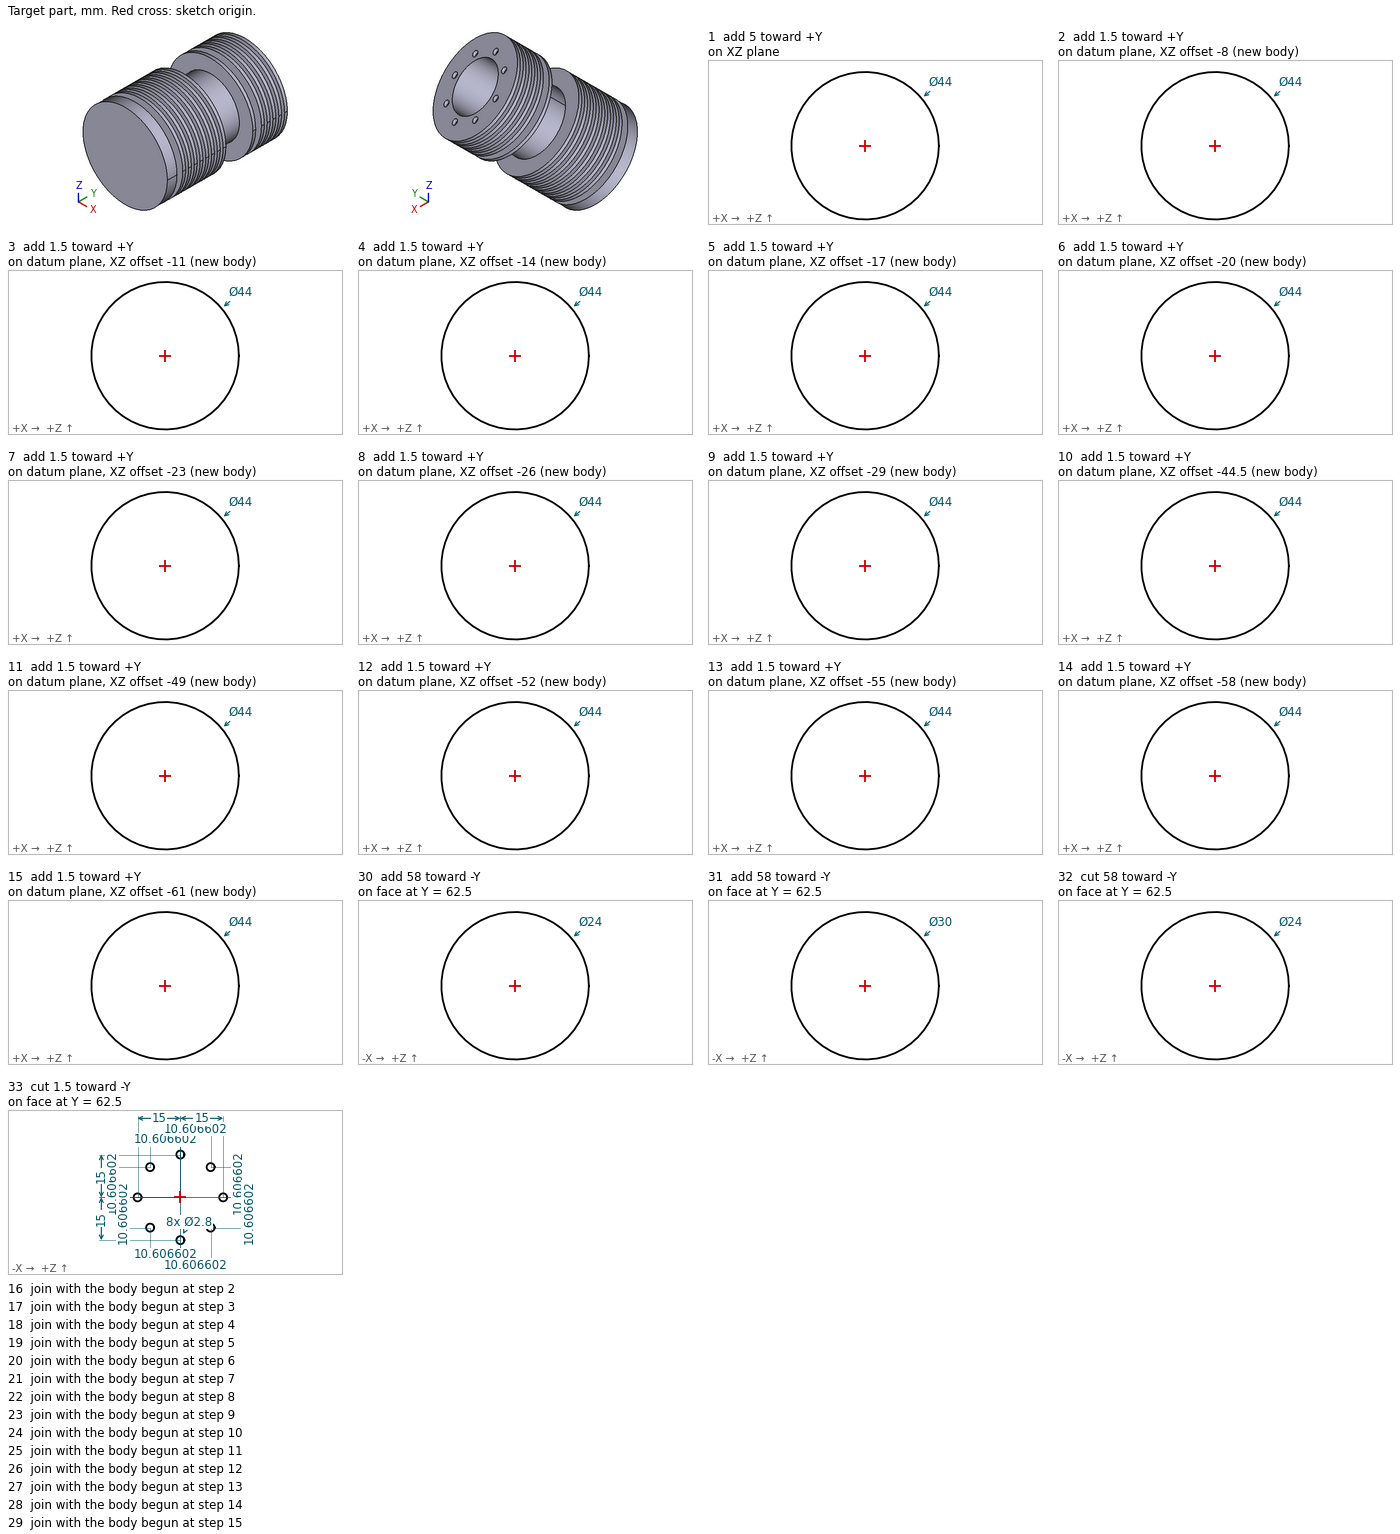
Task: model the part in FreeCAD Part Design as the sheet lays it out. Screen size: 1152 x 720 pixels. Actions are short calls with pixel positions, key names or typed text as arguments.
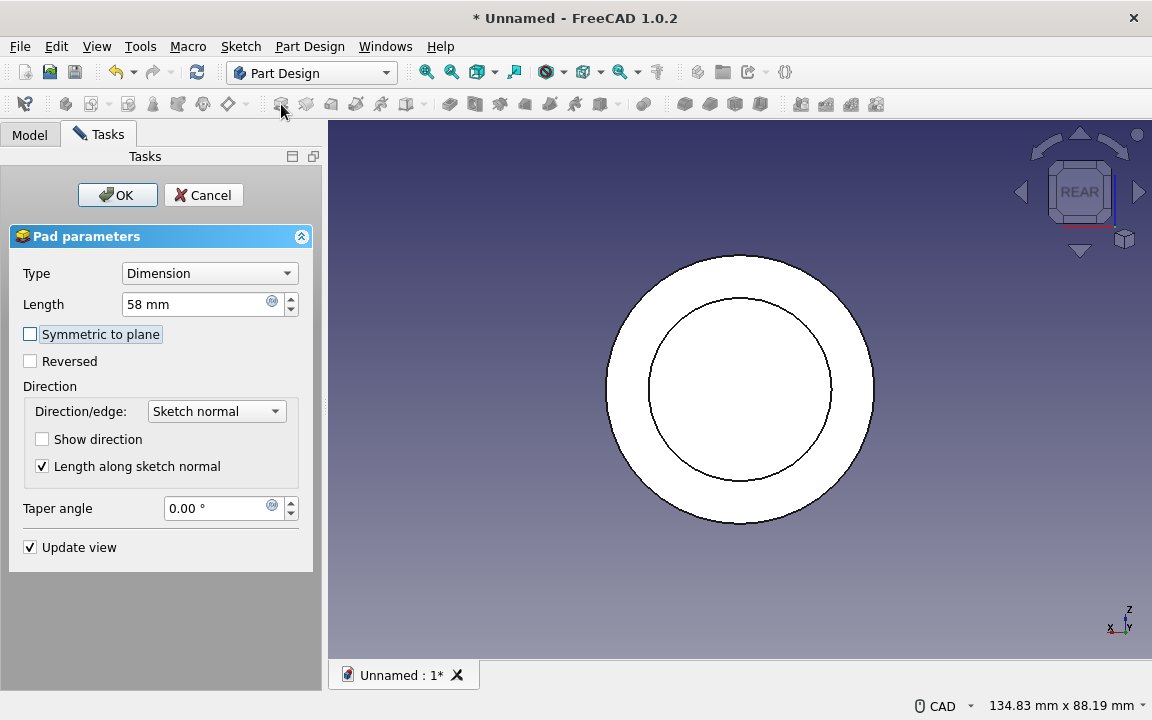
click(31, 361)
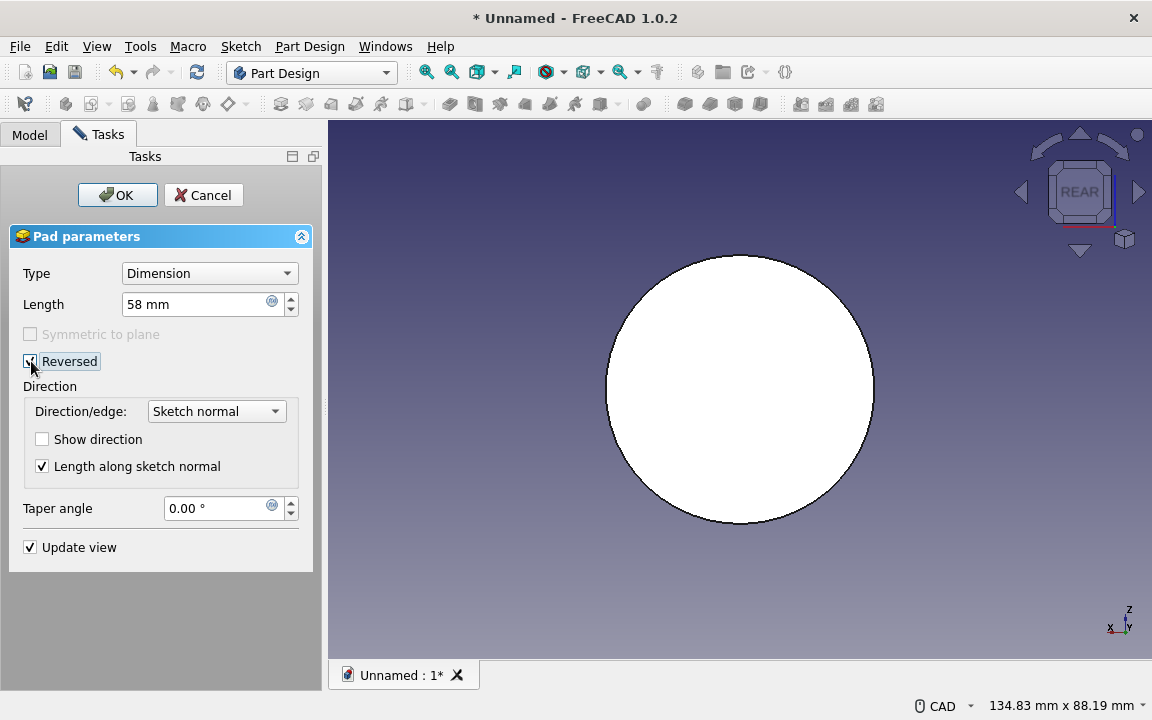
click(118, 195)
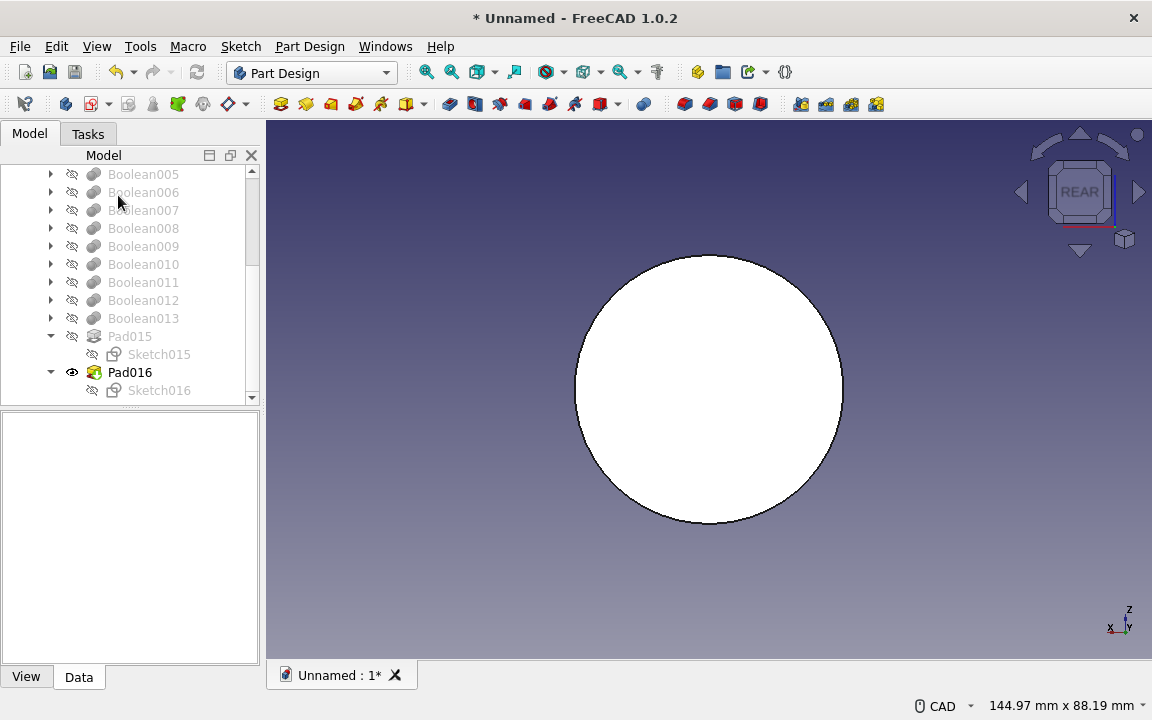
click(709, 389)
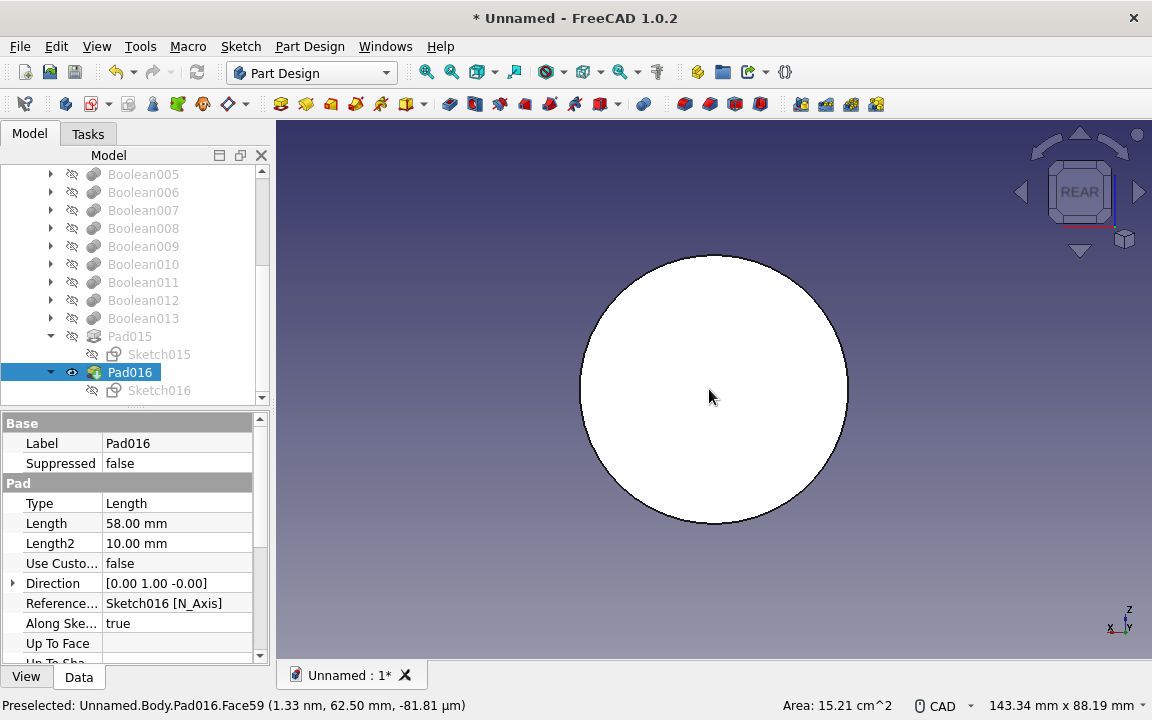
click(90, 104)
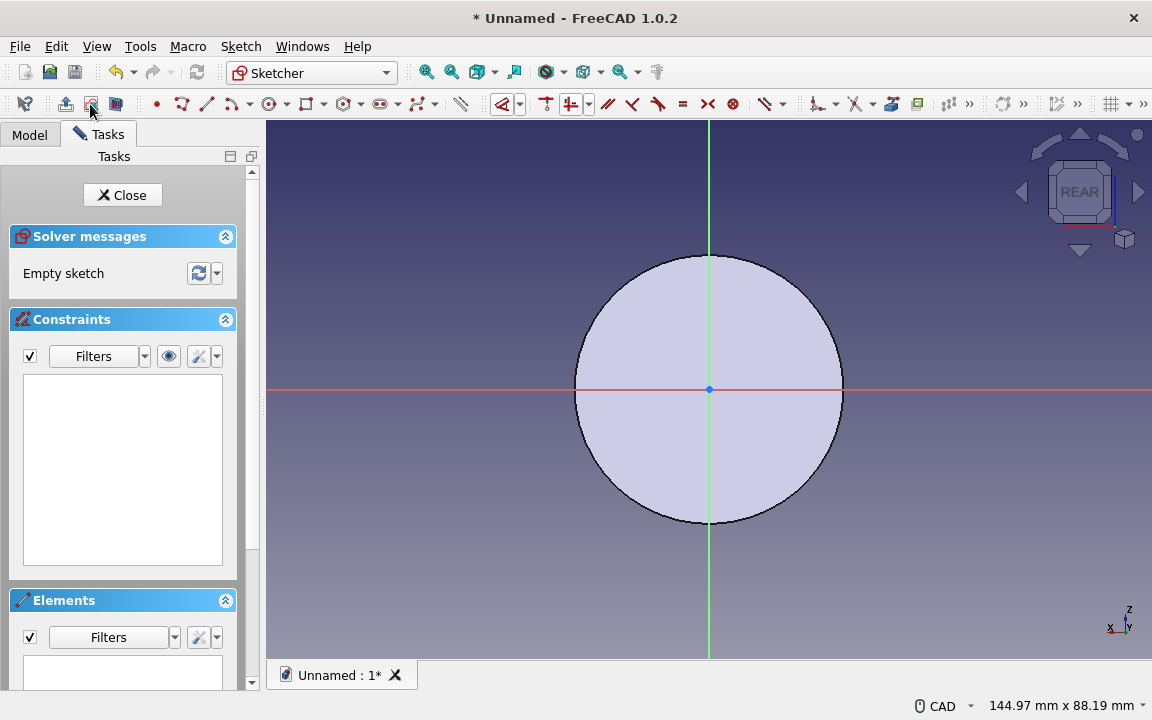
scroll(765, 390, up, 4)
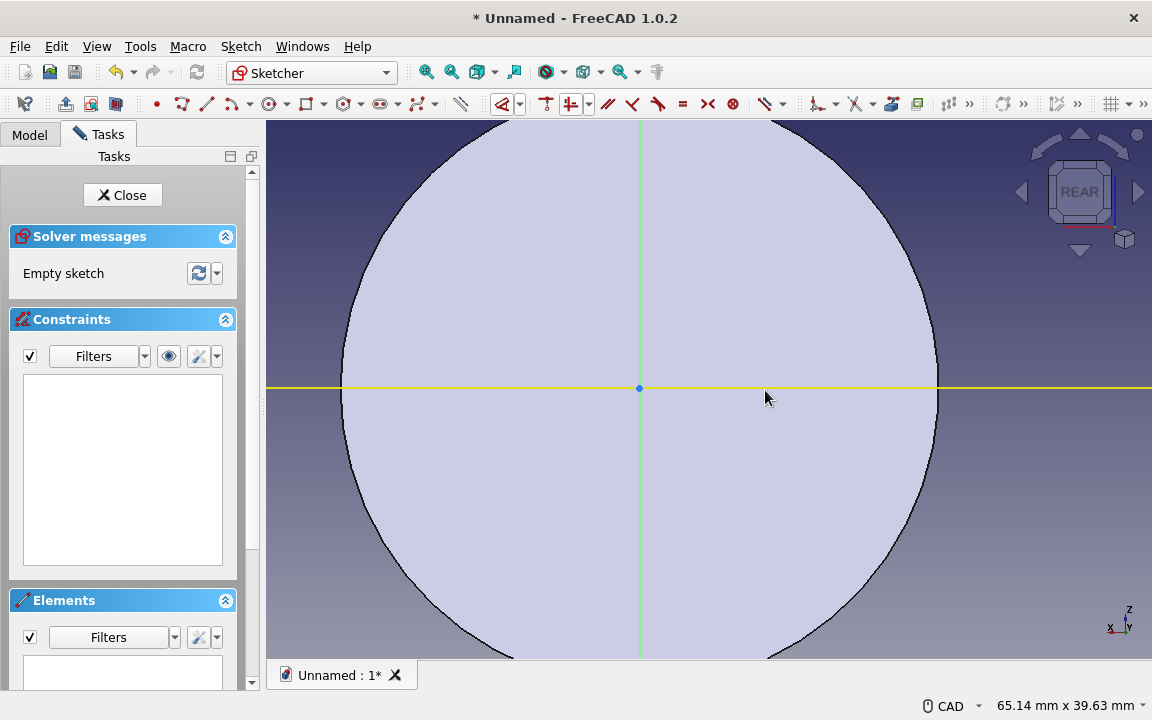
click(268, 104)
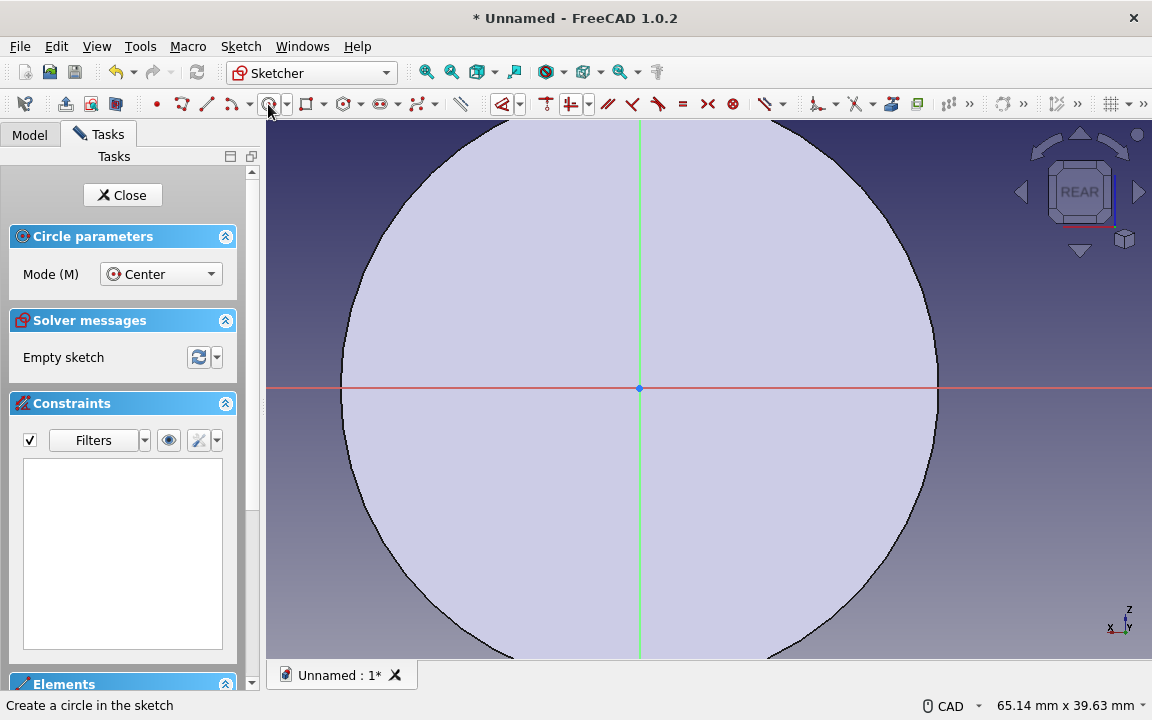
click(640, 388)
click(755, 273)
key(Escape)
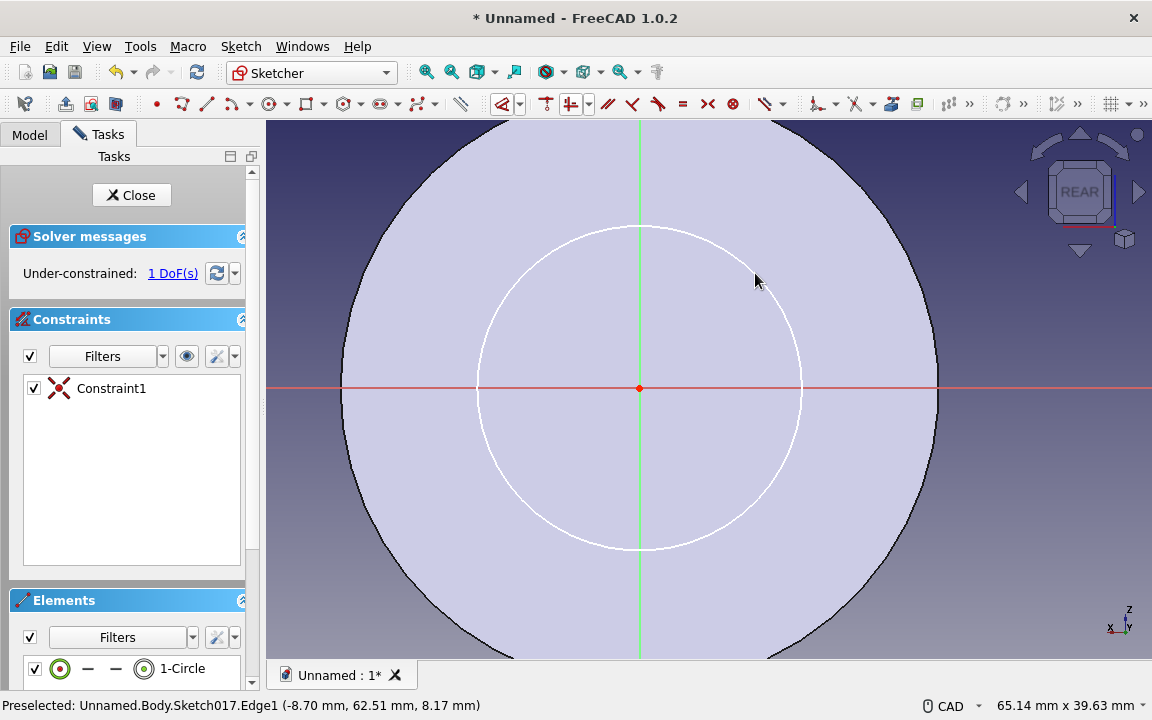
click(754, 273)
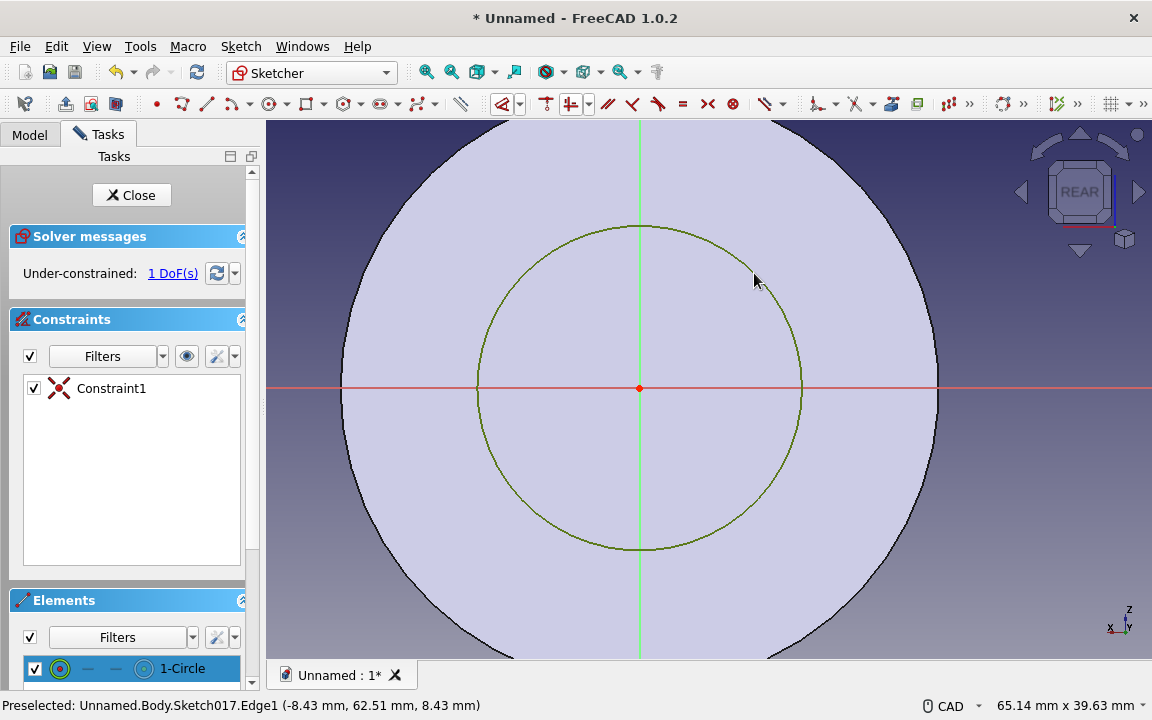
click(520, 104)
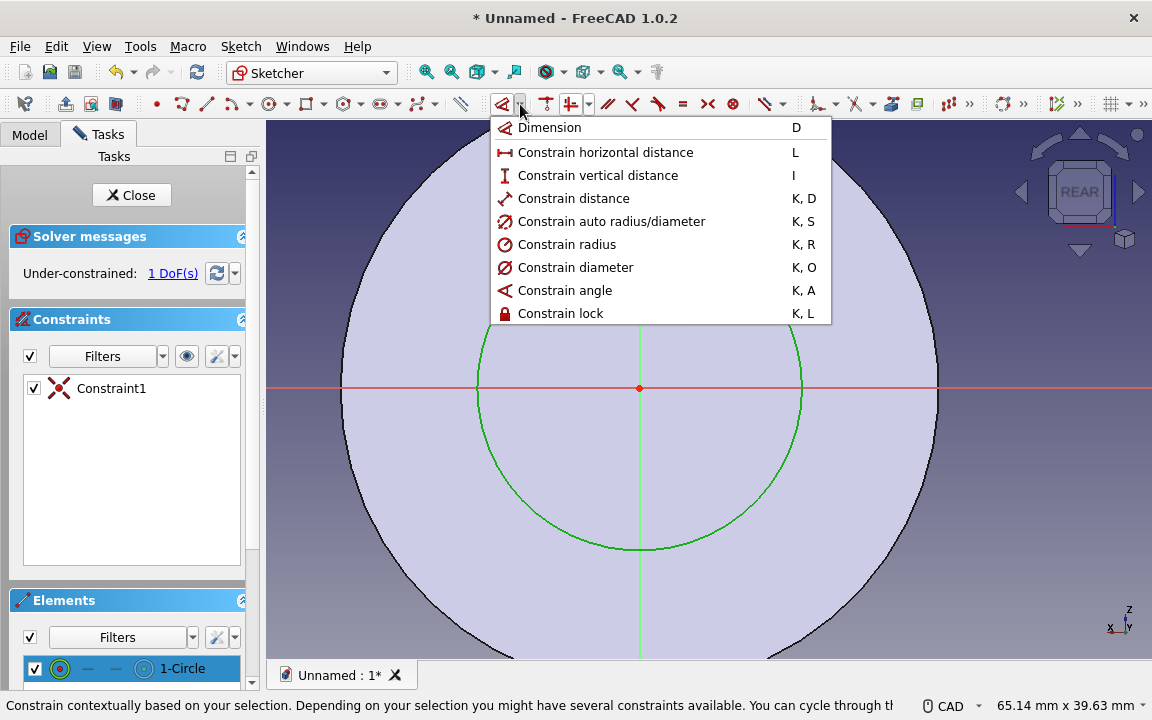
click(661, 268)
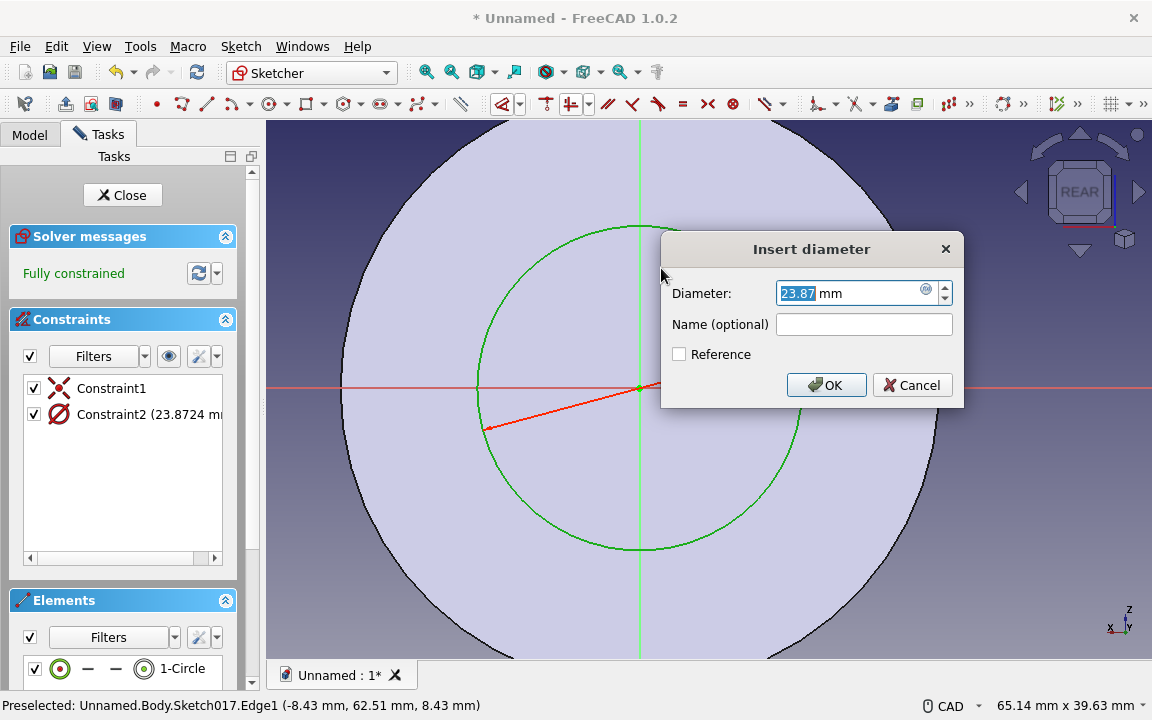
text(24)
key(Return)